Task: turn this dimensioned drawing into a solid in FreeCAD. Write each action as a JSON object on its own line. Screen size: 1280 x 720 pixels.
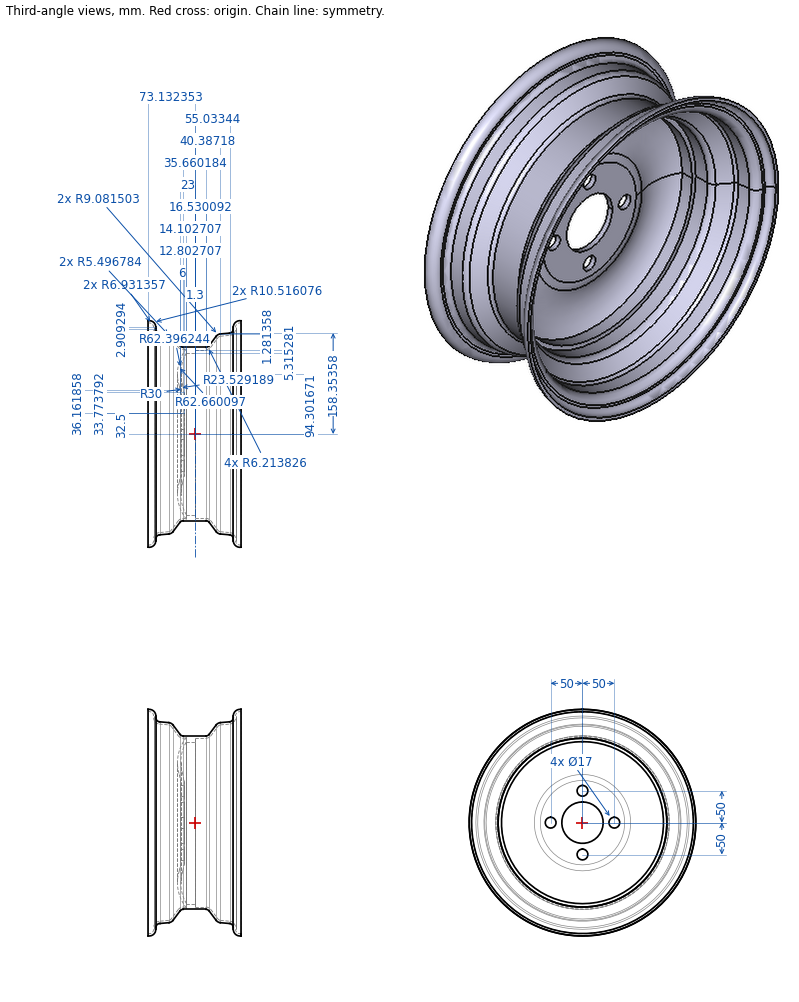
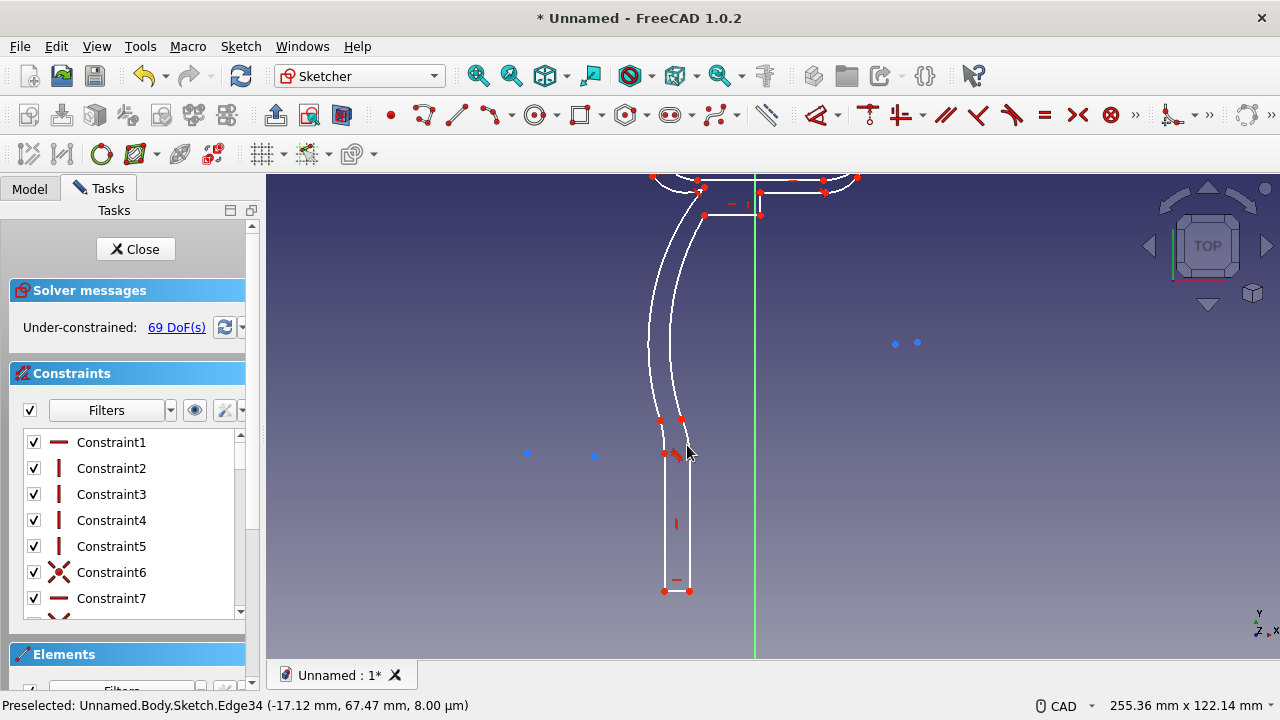
{"action": "scroll", "coordinate": [663, 458], "scroll_direction": "down", "scroll_amount": 4}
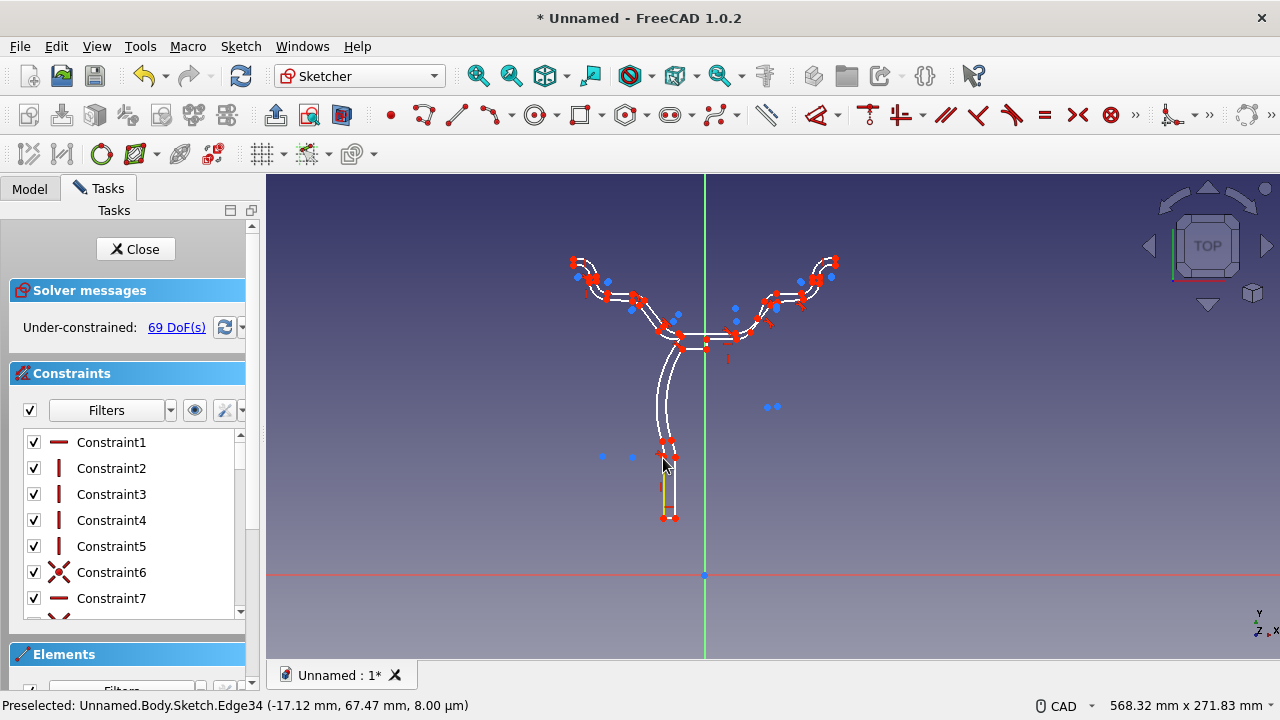
{"action": "scroll", "coordinate": [716, 339], "scroll_direction": "up", "scroll_amount": 5}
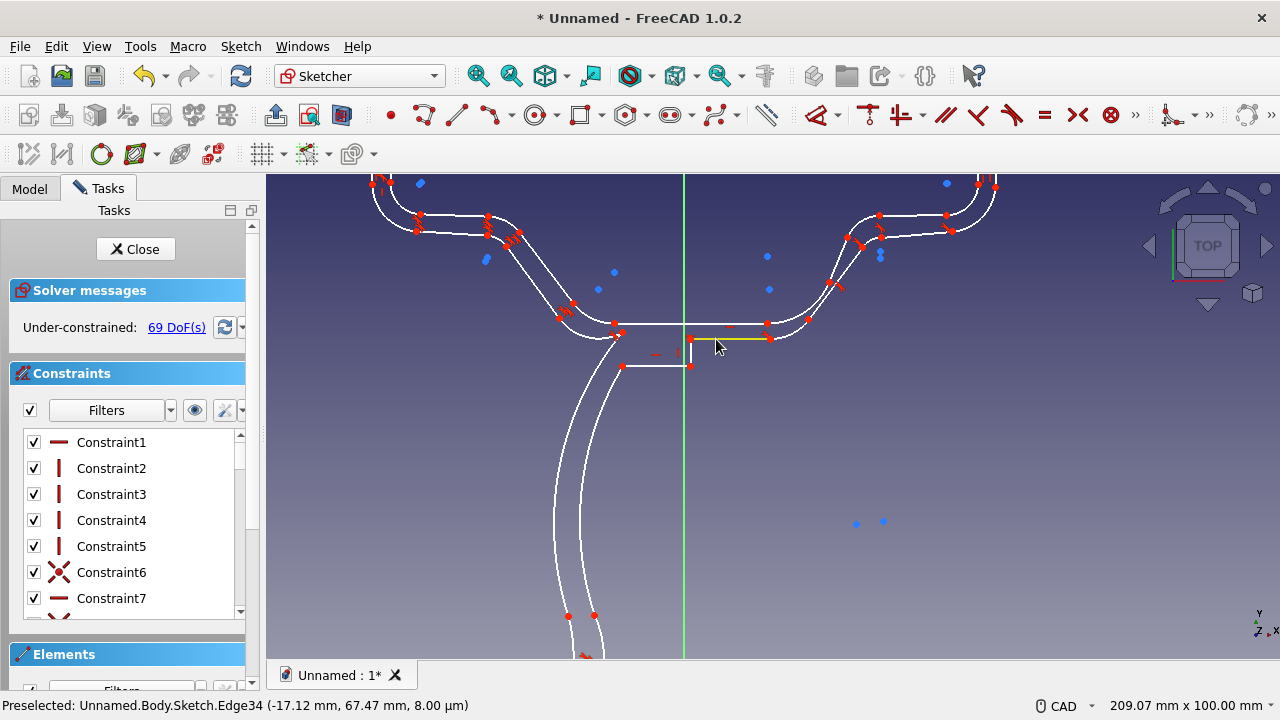
{"action": "left_click", "coordinate": [715, 339]}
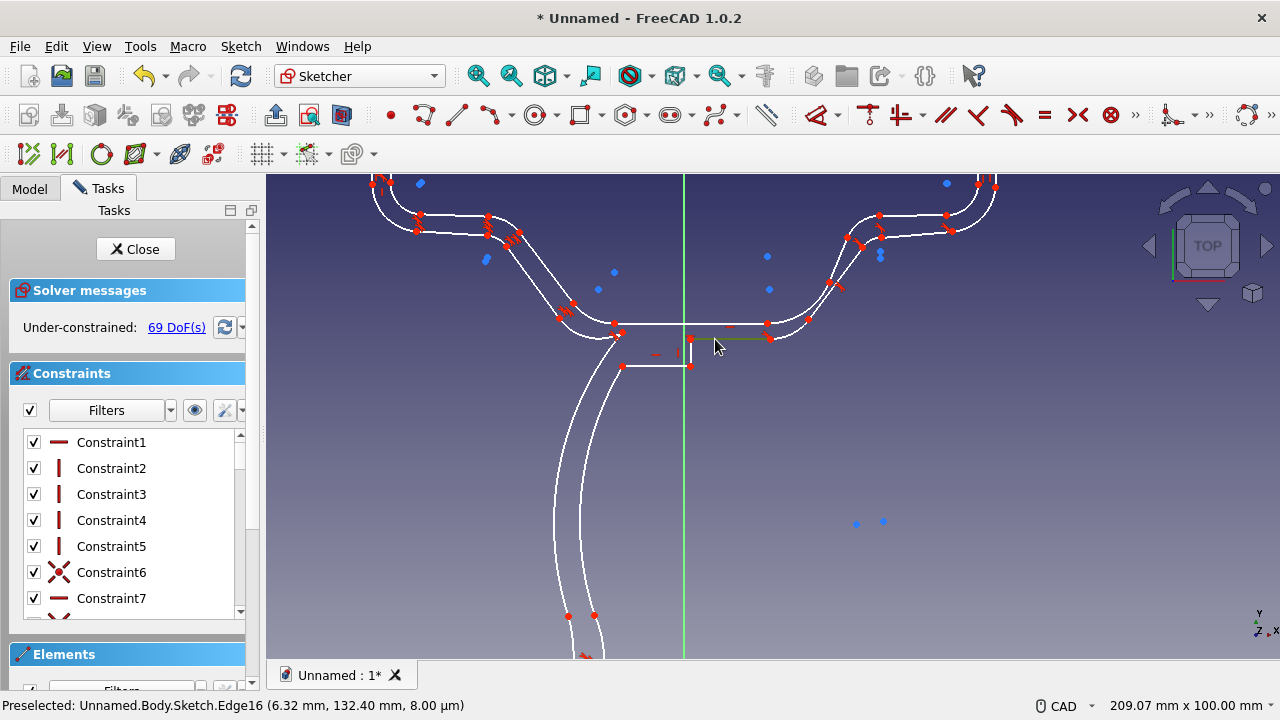
{"action": "left_click", "coordinate": [784, 337]}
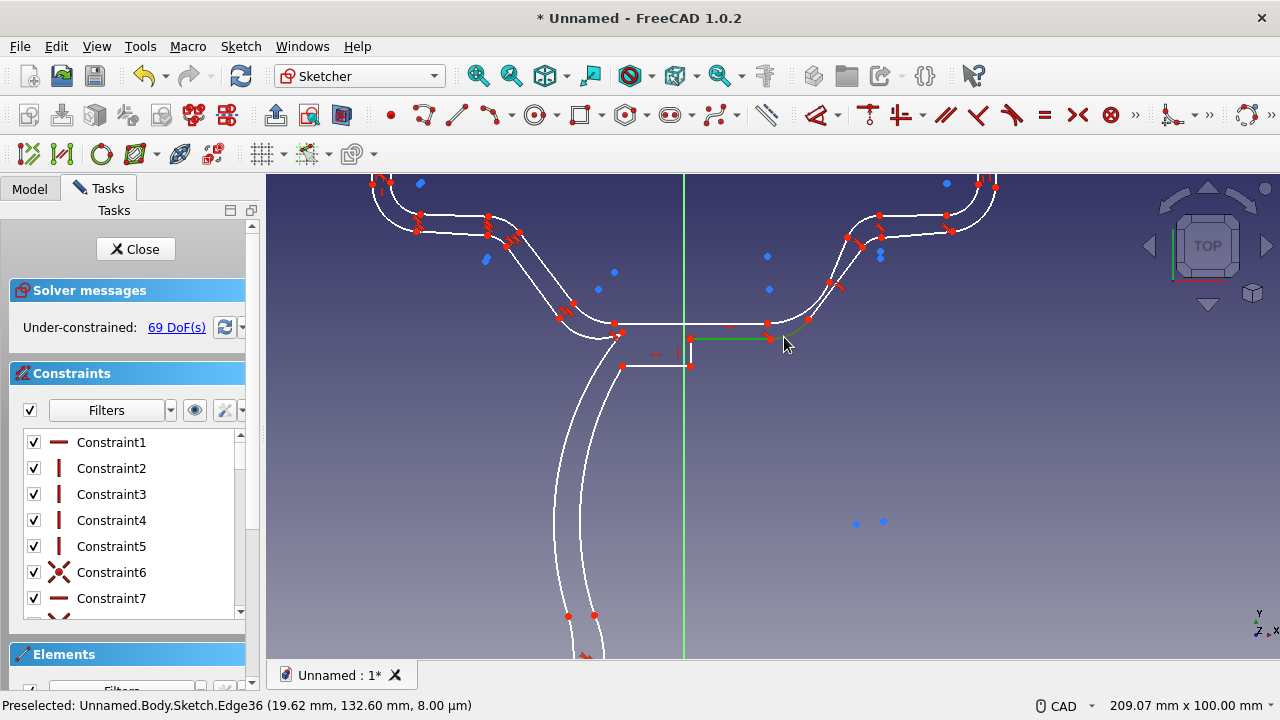
{"action": "left_click", "coordinate": [1012, 116]}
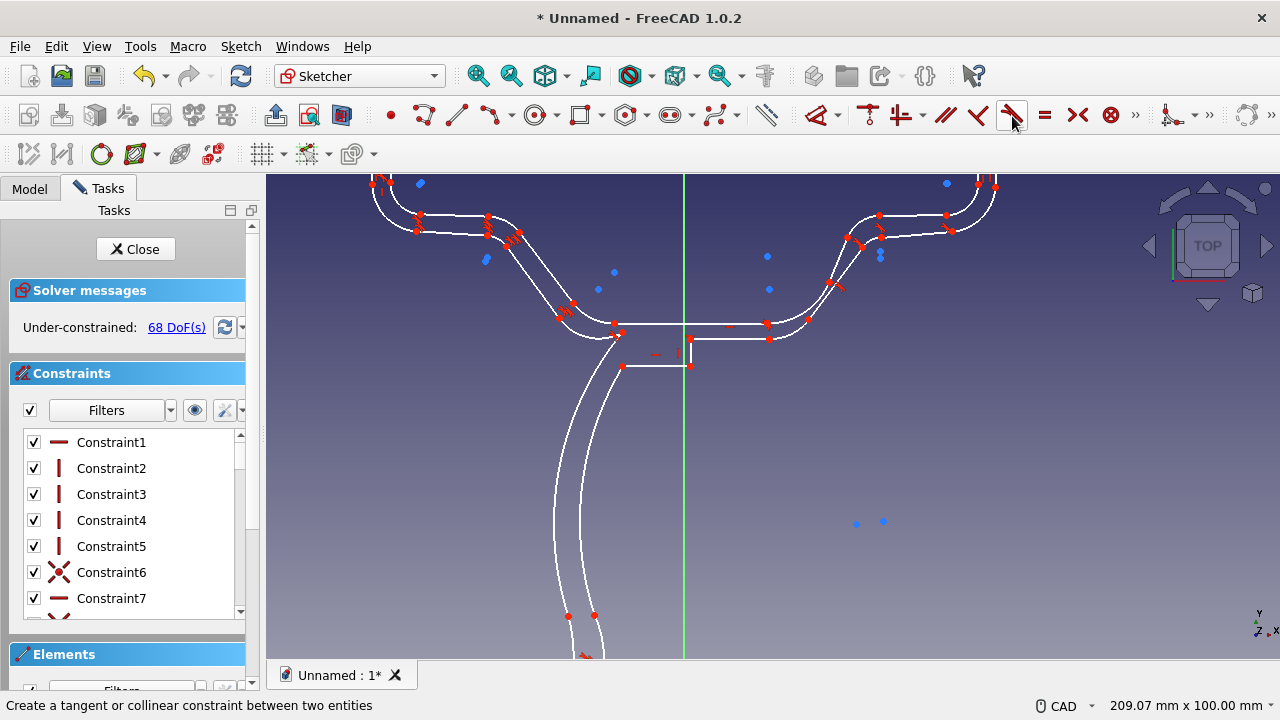
{"action": "scroll", "coordinate": [847, 270], "scroll_direction": "up", "scroll_amount": 2}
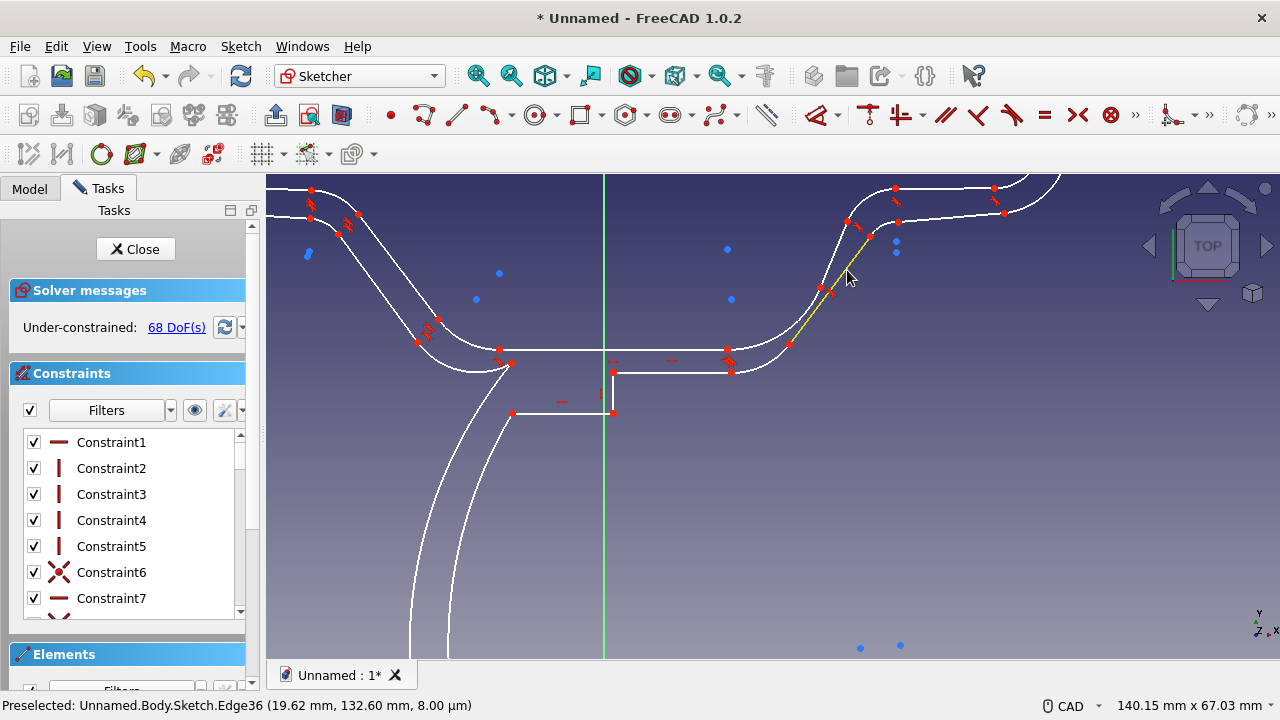
{"action": "left_click", "coordinate": [846, 269]}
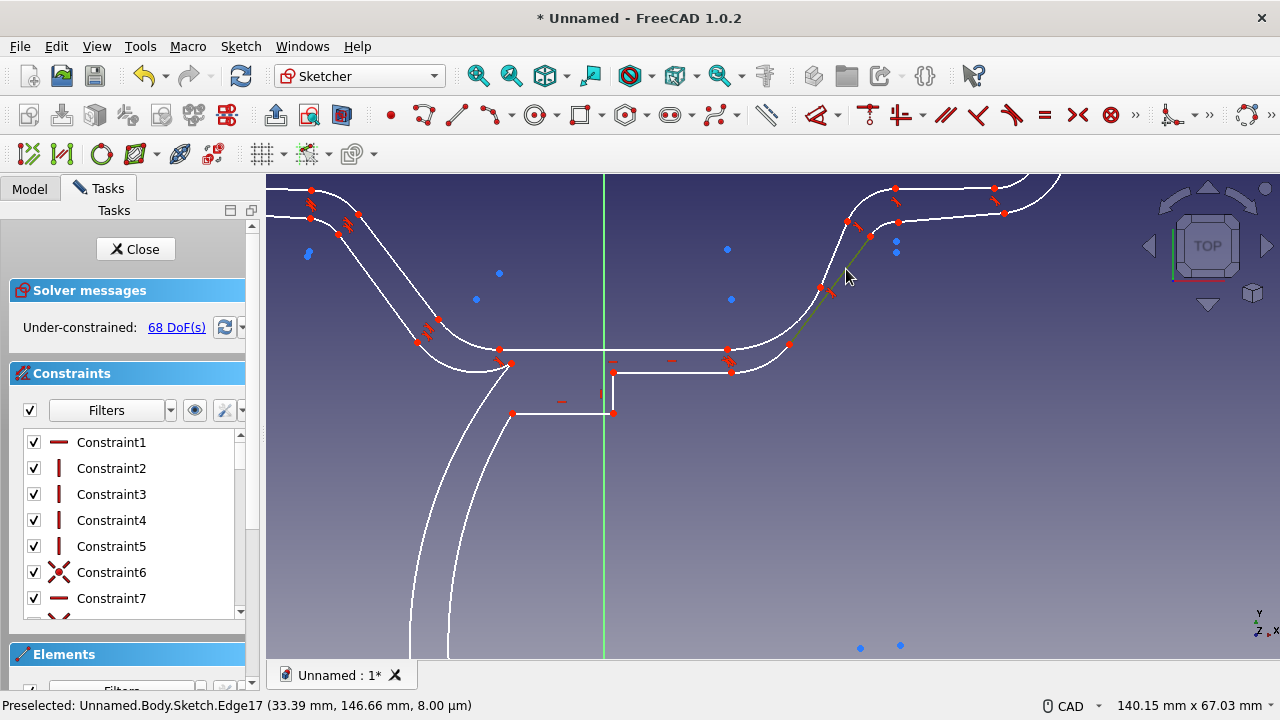
{"action": "left_click", "coordinate": [752, 370]}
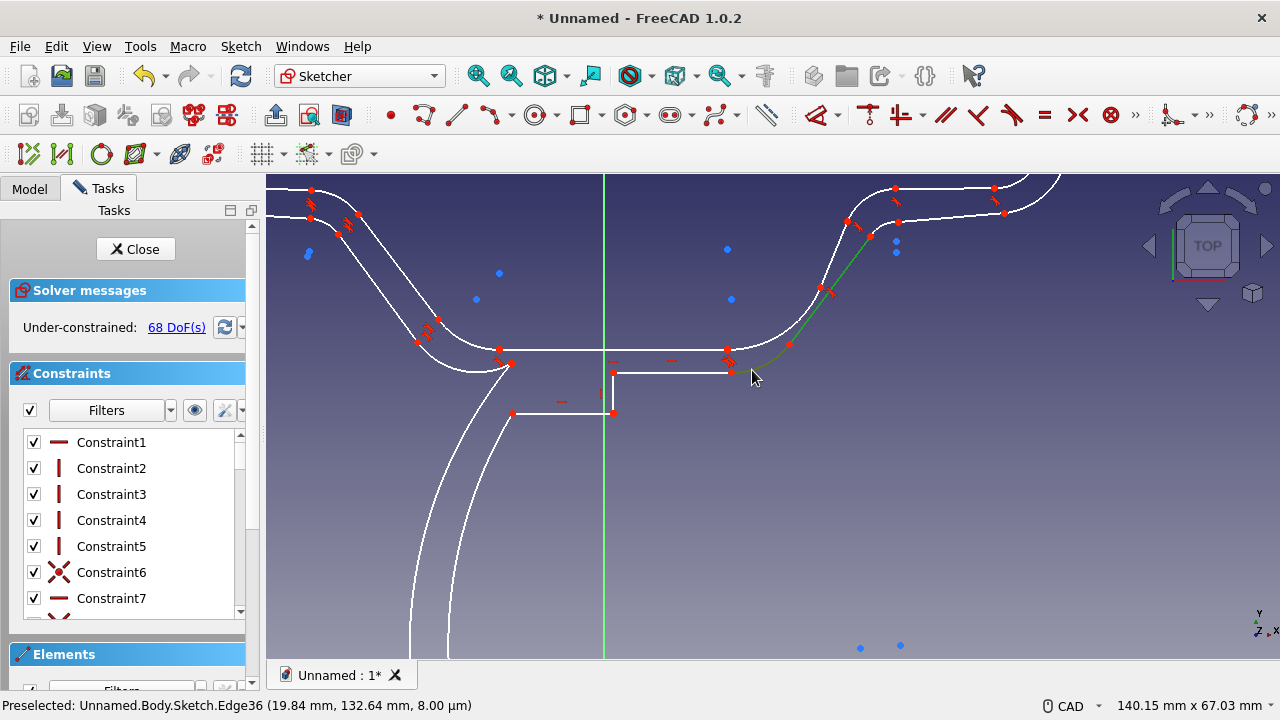
{"action": "key", "text": "t"}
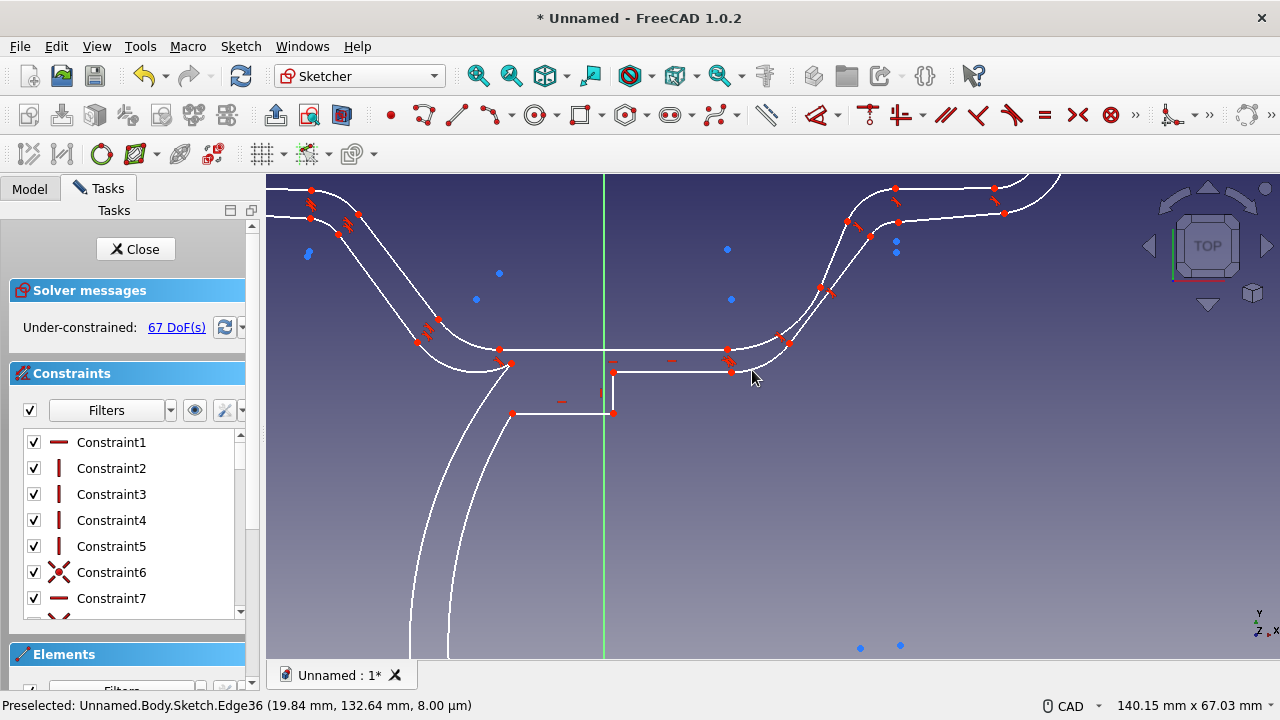
{"action": "left_click", "coordinate": [846, 269]}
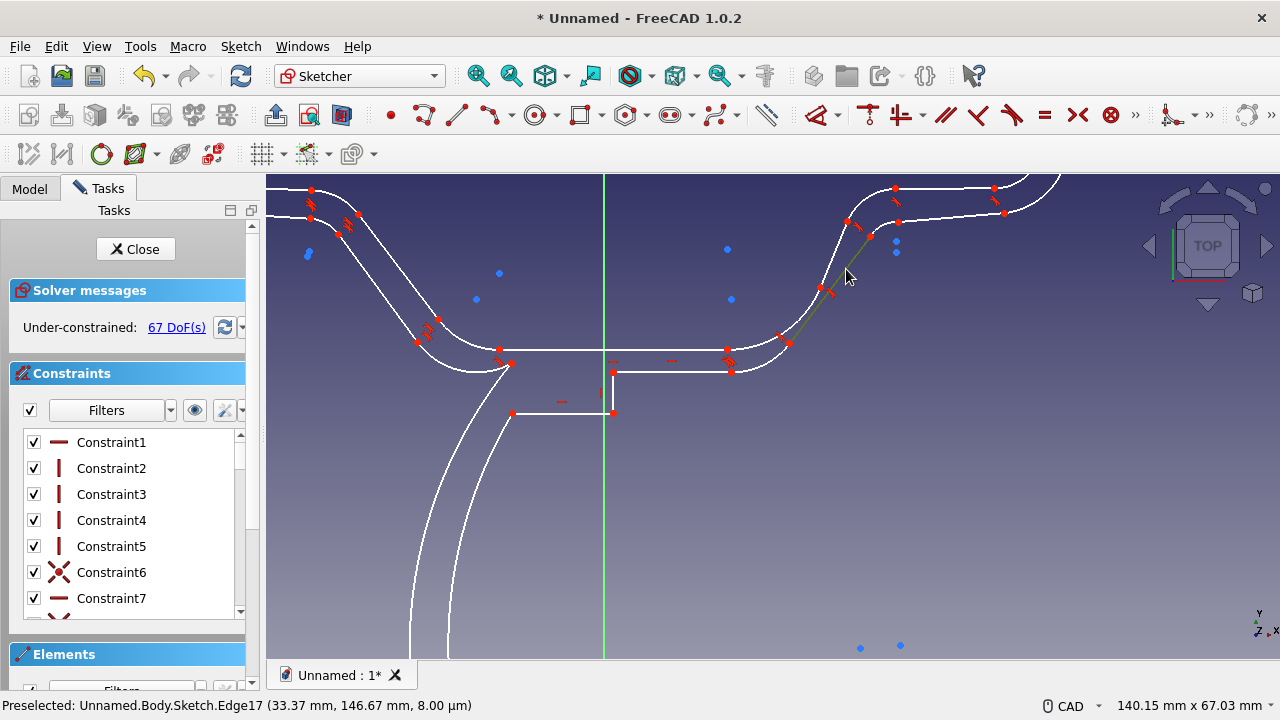
{"action": "scroll", "coordinate": [889, 223], "scroll_direction": "up", "scroll_amount": 2}